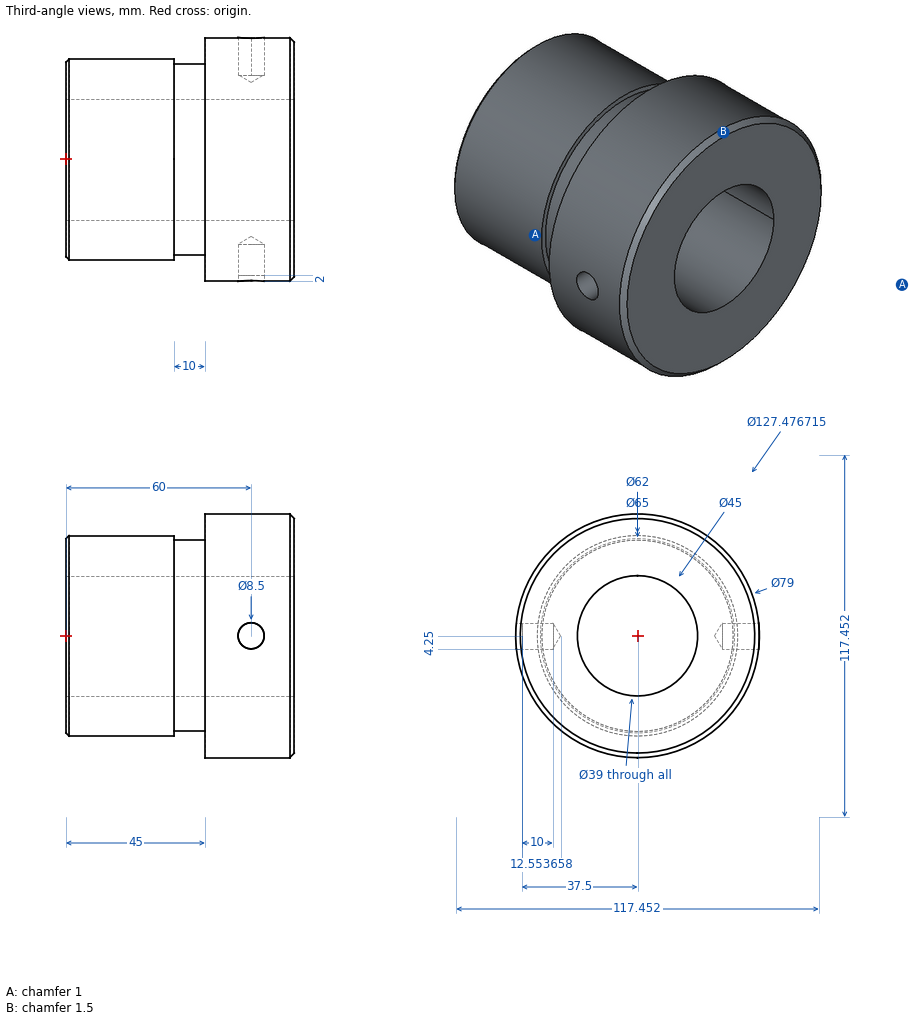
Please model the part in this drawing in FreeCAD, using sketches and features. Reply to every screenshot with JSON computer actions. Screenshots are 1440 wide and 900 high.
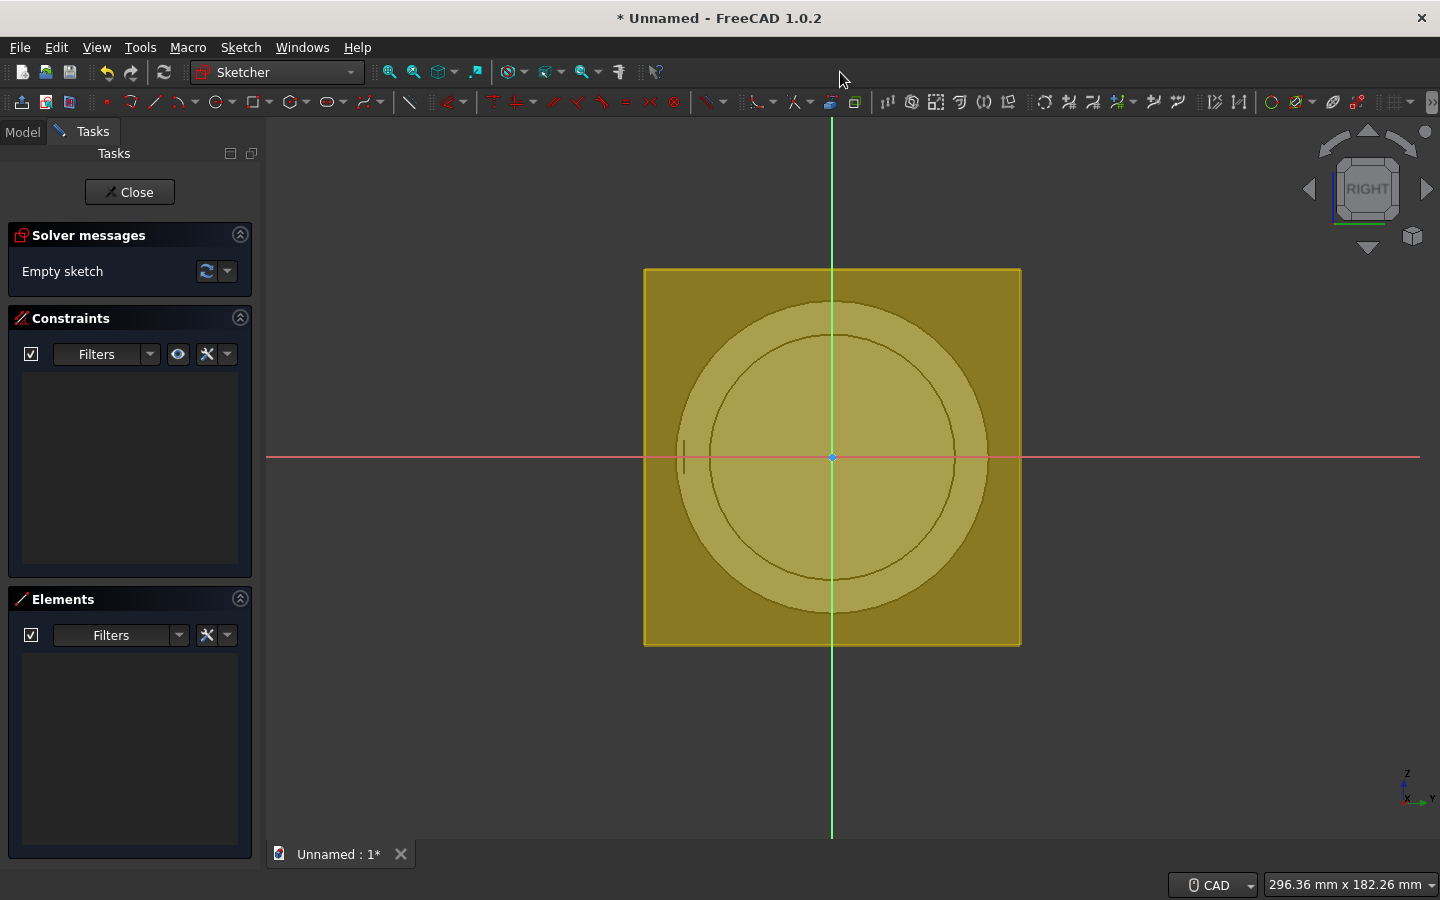
{"action": "scroll", "coordinate": [702, 465], "scroll_direction": "up", "scroll_amount": 13}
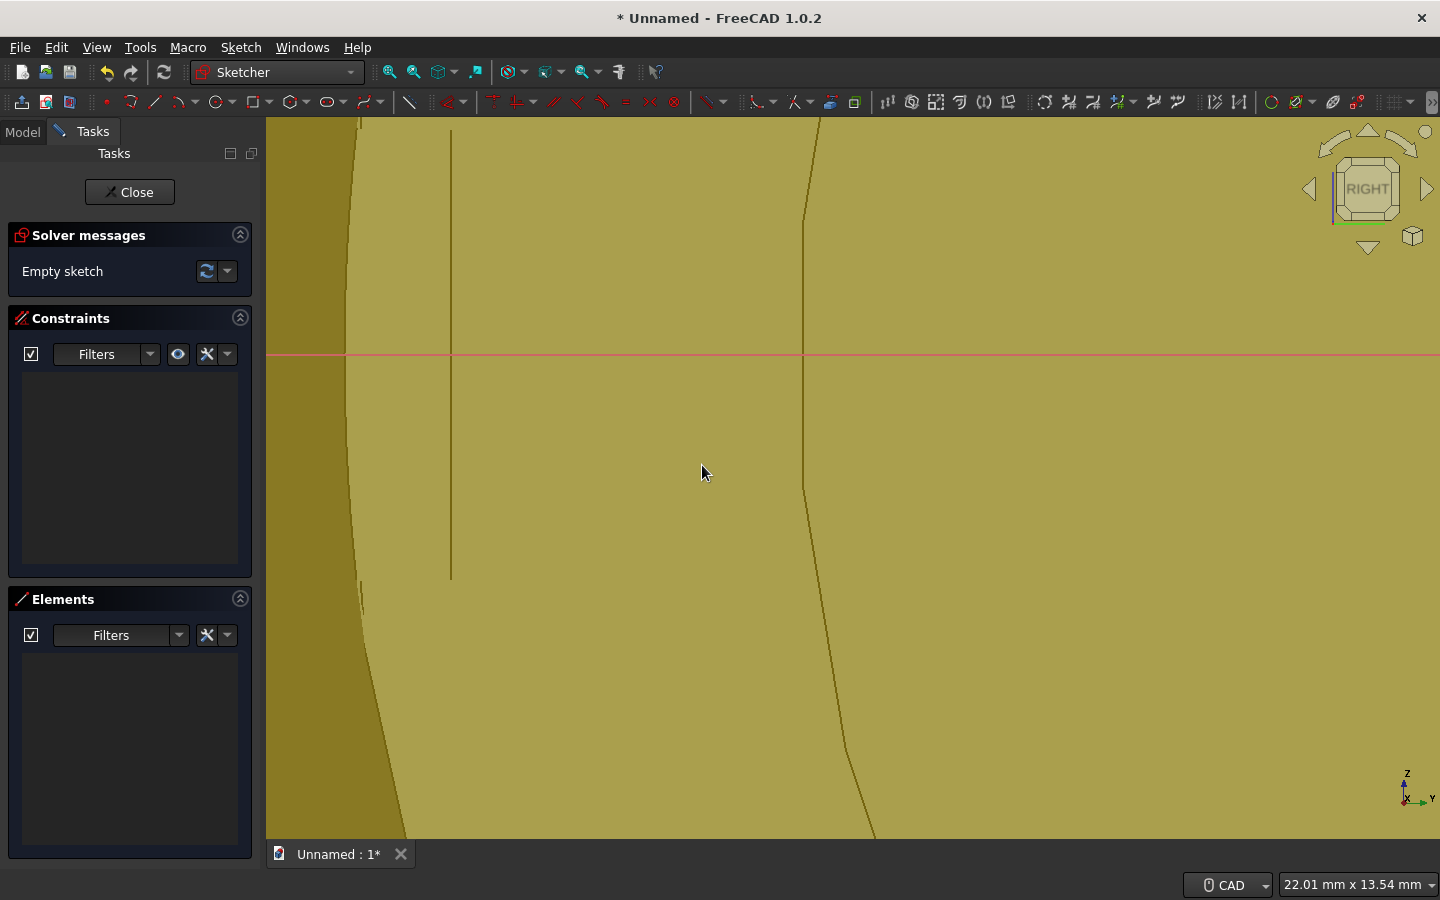
{"action": "key", "text": "g m"}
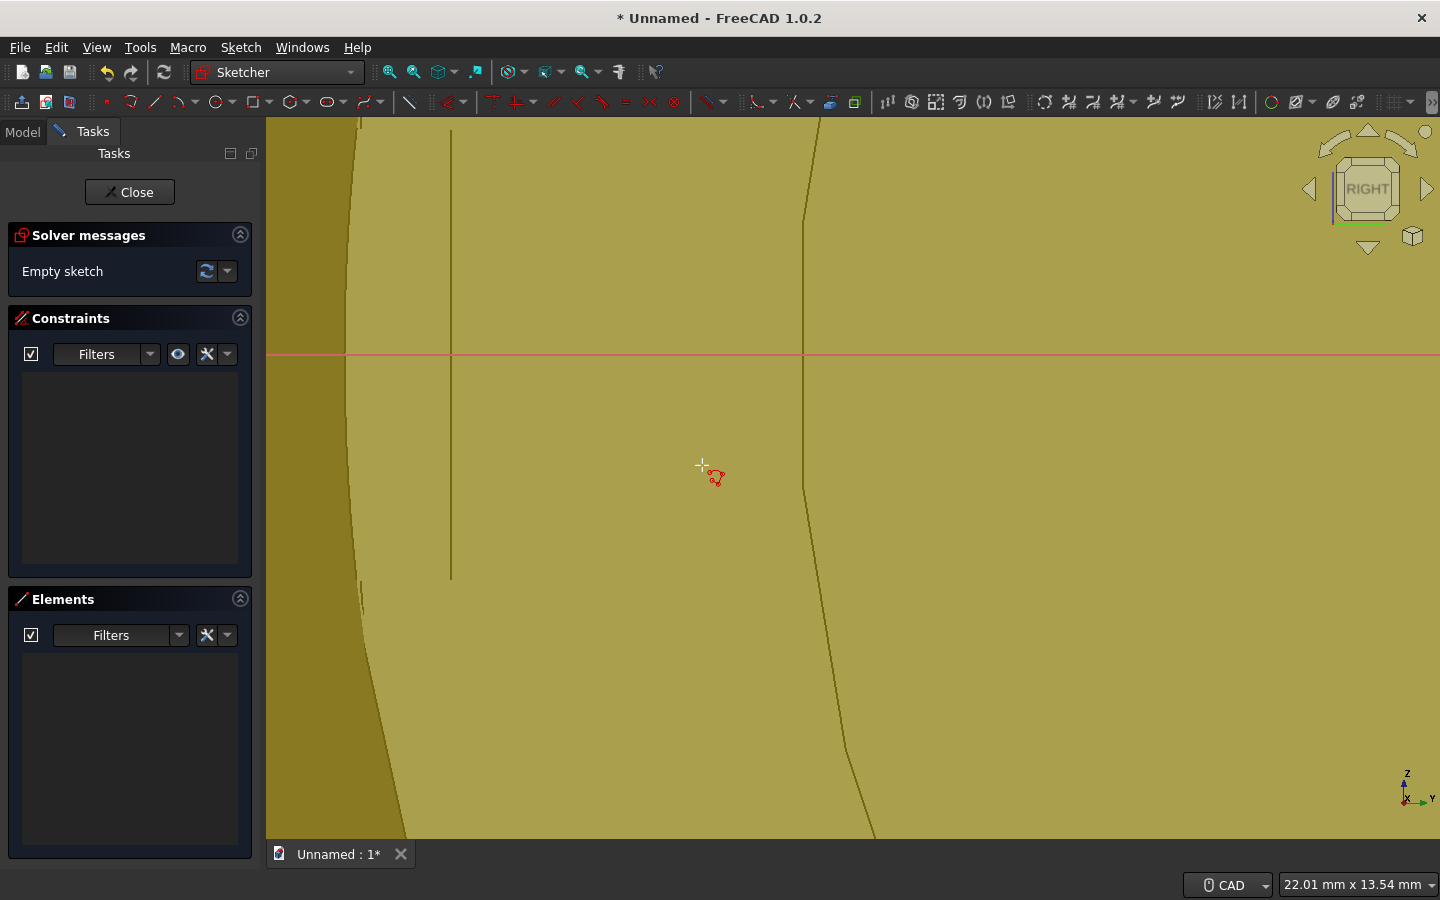
{"action": "left_click", "coordinate": [1121, 355]}
{"action": "left_click", "coordinate": [451, 364]}
{"action": "left_click", "coordinate": [451, 582]}
{"action": "left_click", "coordinate": [985, 582]}
{"action": "left_click", "coordinate": [1121, 355]}
{"action": "key", "text": "Escape"}
{"action": "key", "text": "Escape"}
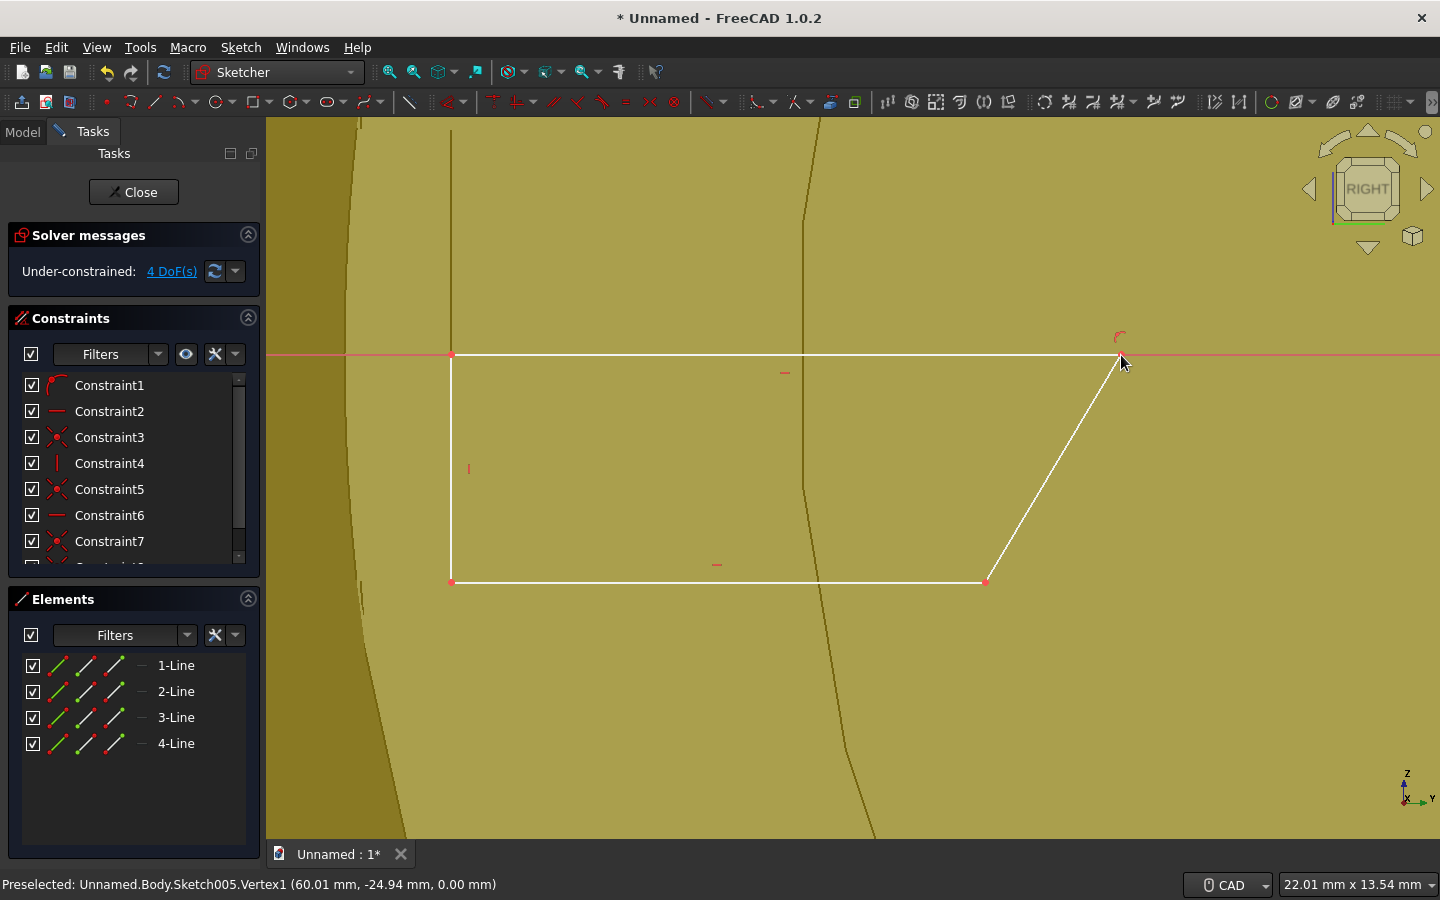
{"action": "key", "text": "d"}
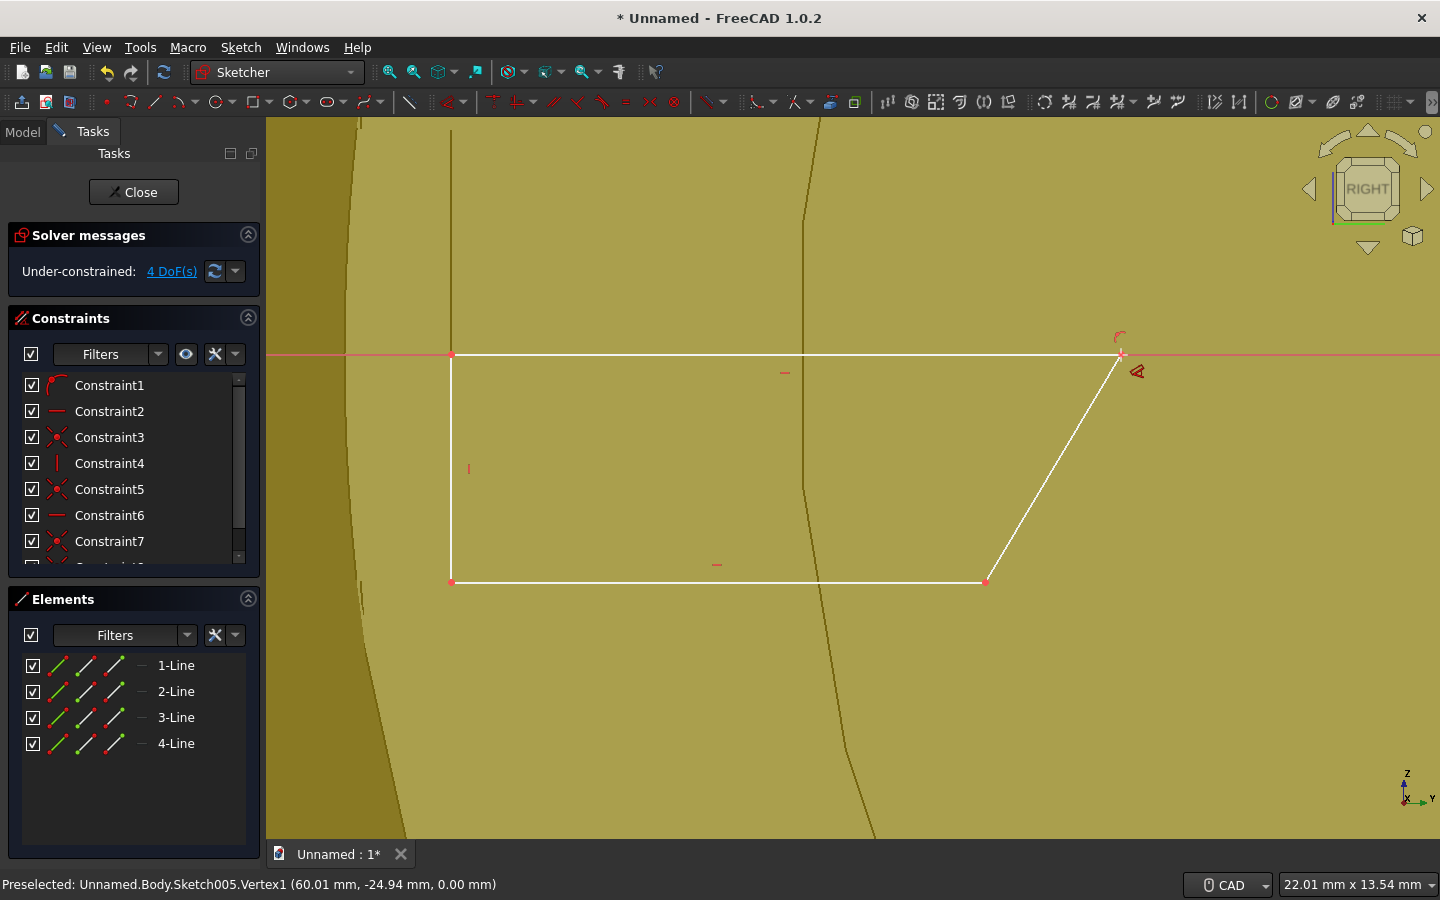
{"action": "left_click", "coordinate": [611, 583]}
{"action": "left_click", "coordinate": [718, 617]}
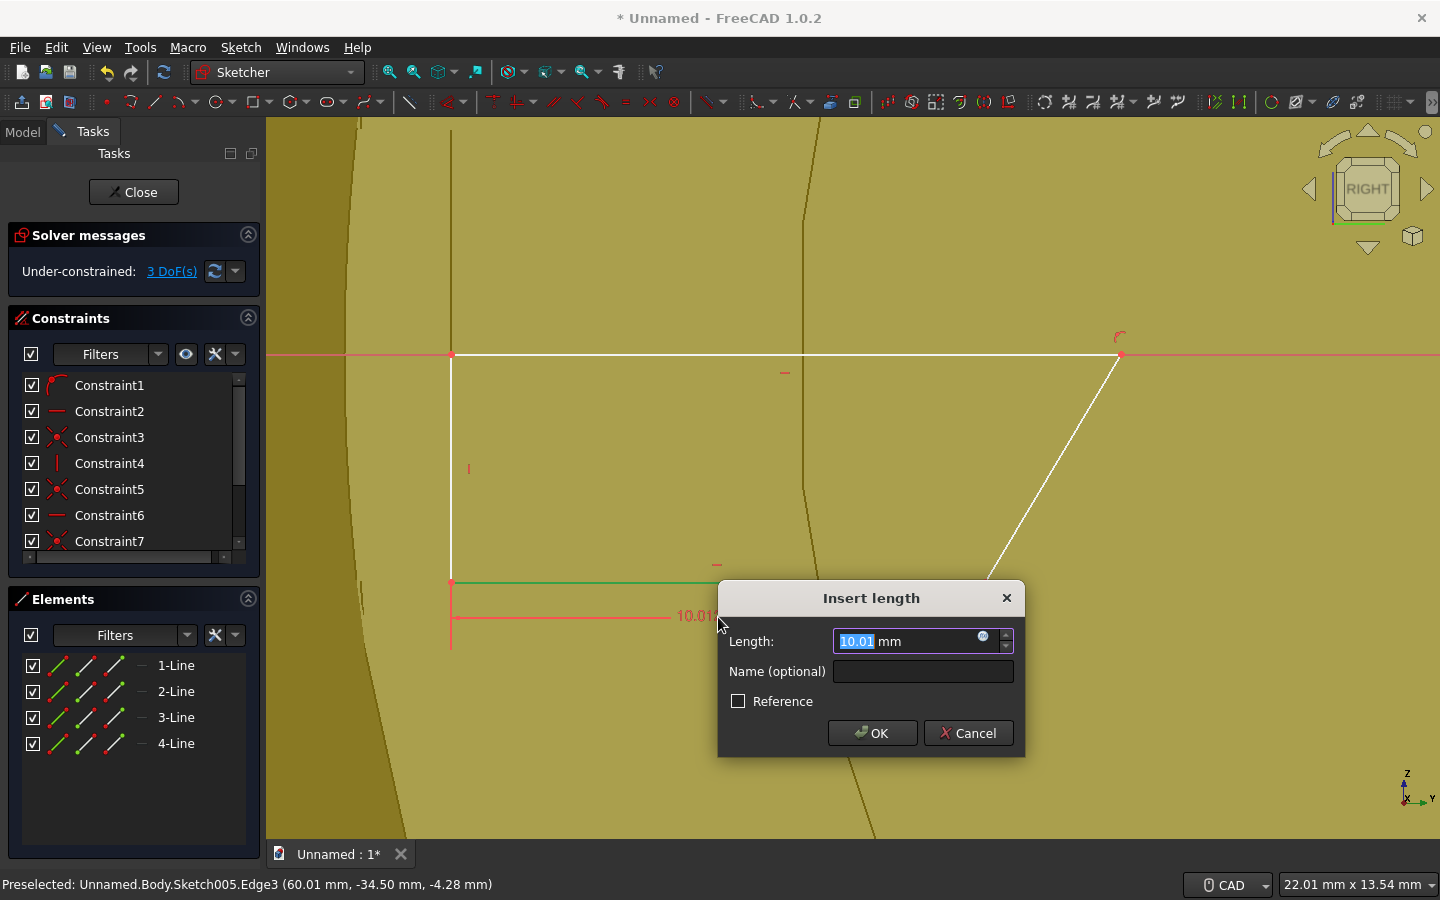
{"action": "type", "text": "10"}
{"action": "key", "text": "Return"}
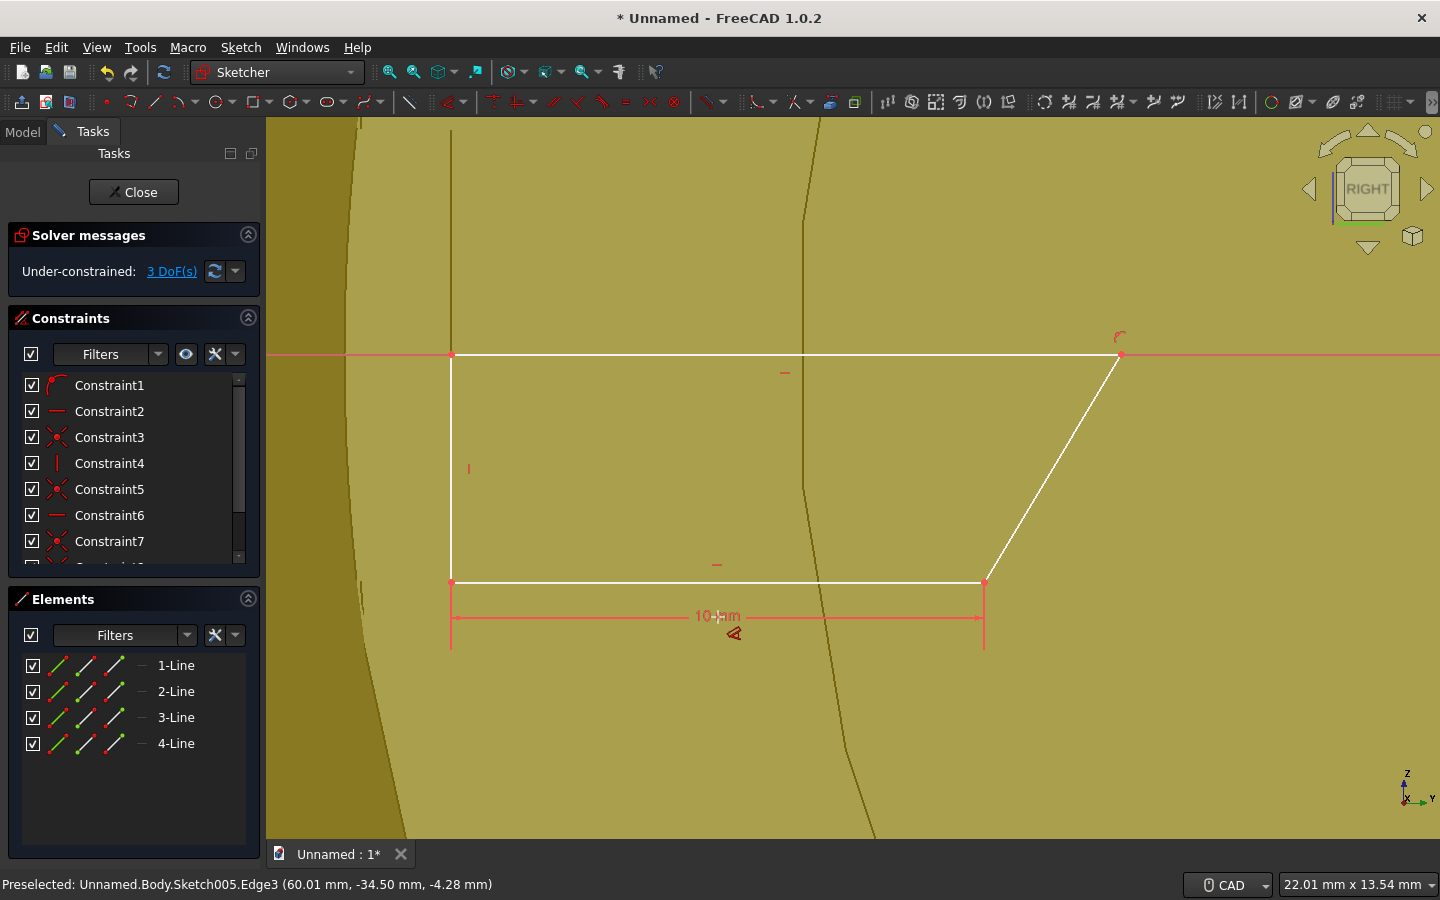
{"action": "left_click", "coordinate": [451, 423]}
{"action": "left_click", "coordinate": [417, 469]}